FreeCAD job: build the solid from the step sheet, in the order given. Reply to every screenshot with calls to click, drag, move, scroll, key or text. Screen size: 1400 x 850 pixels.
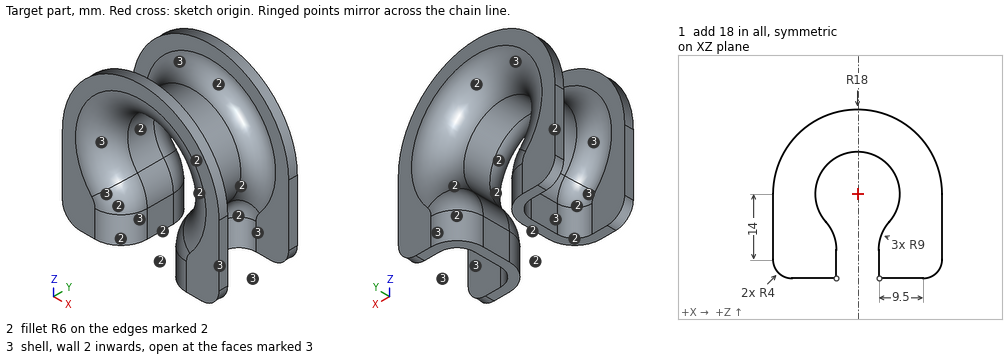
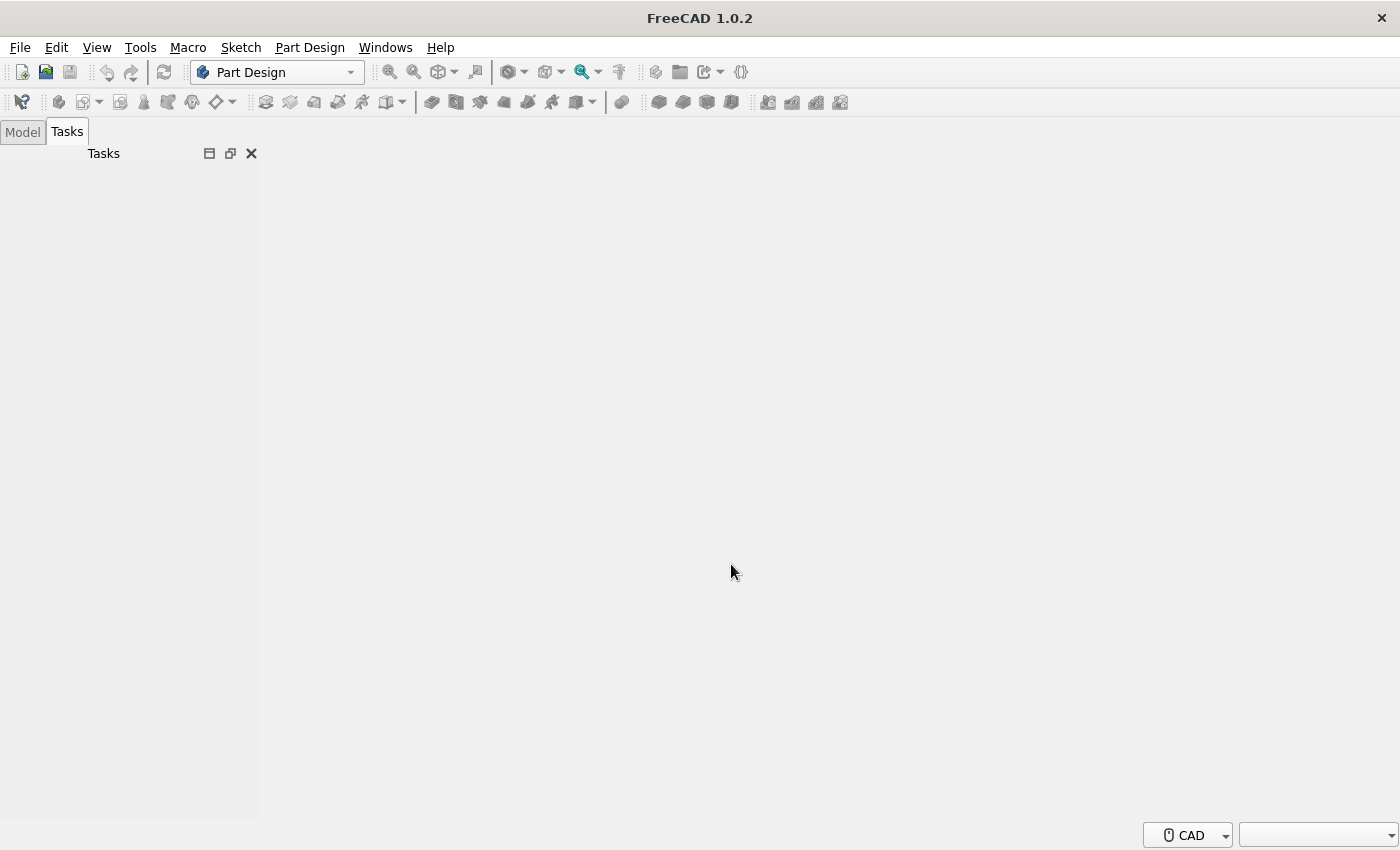
click(22, 72)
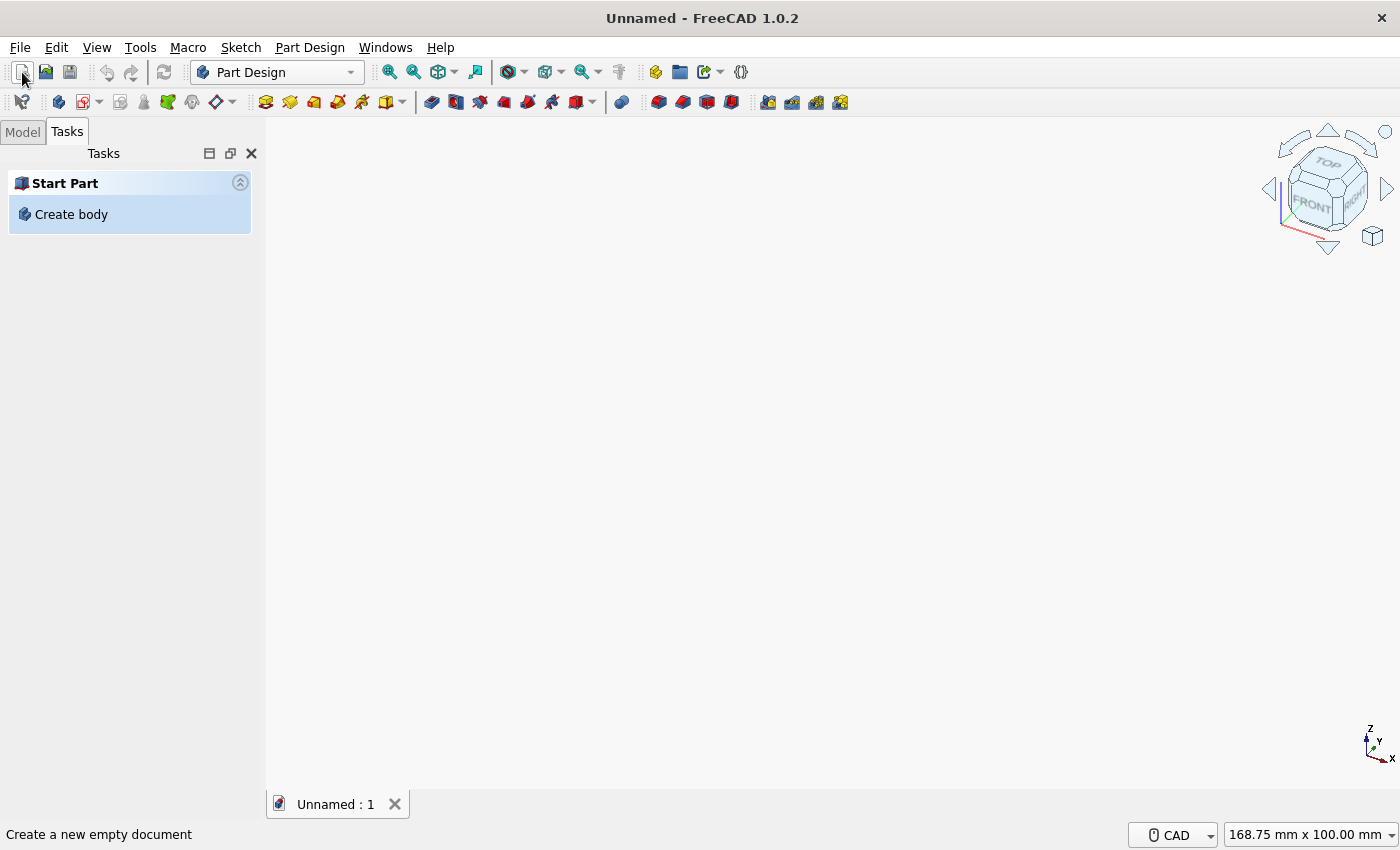
click(84, 102)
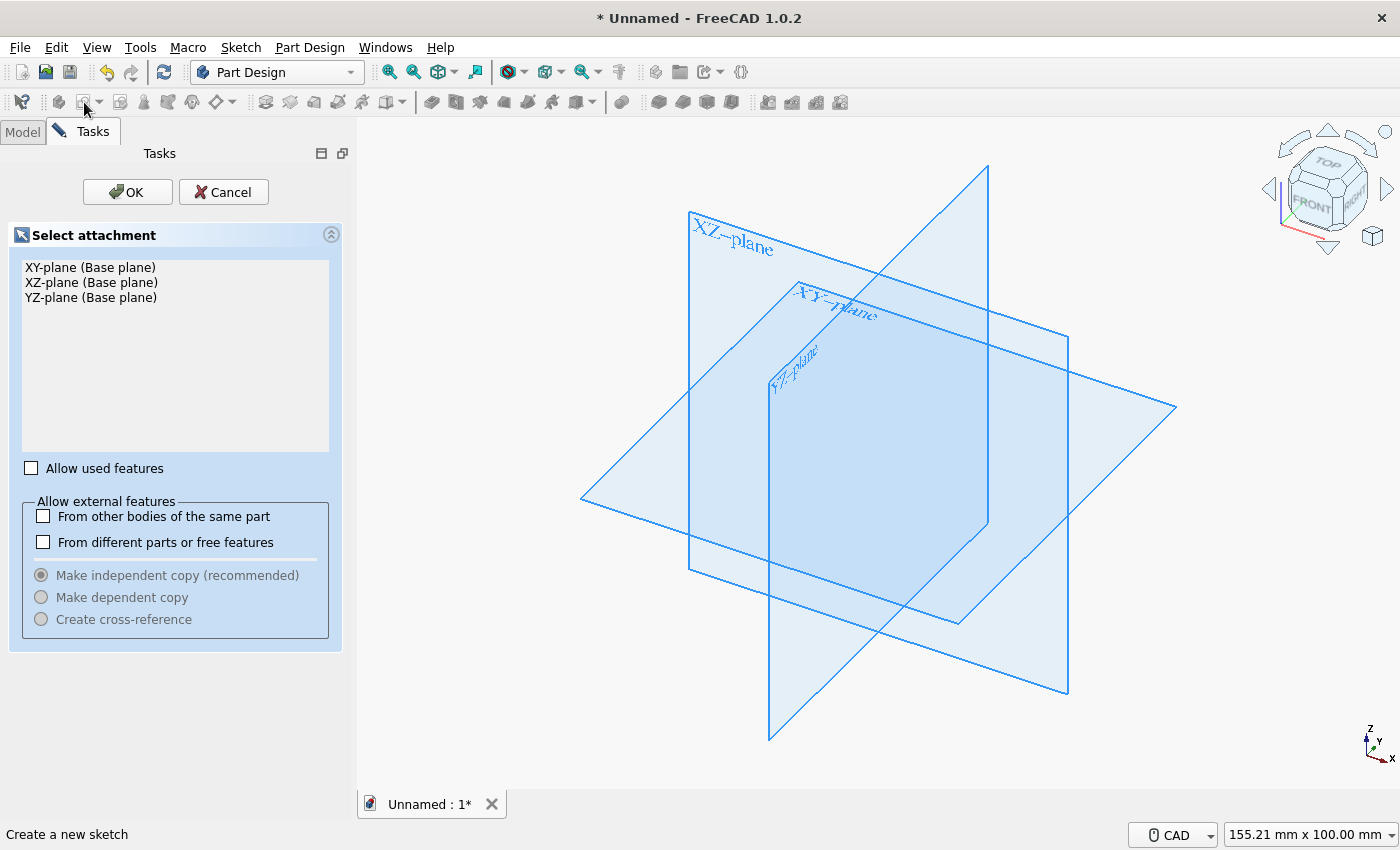
click(82, 282)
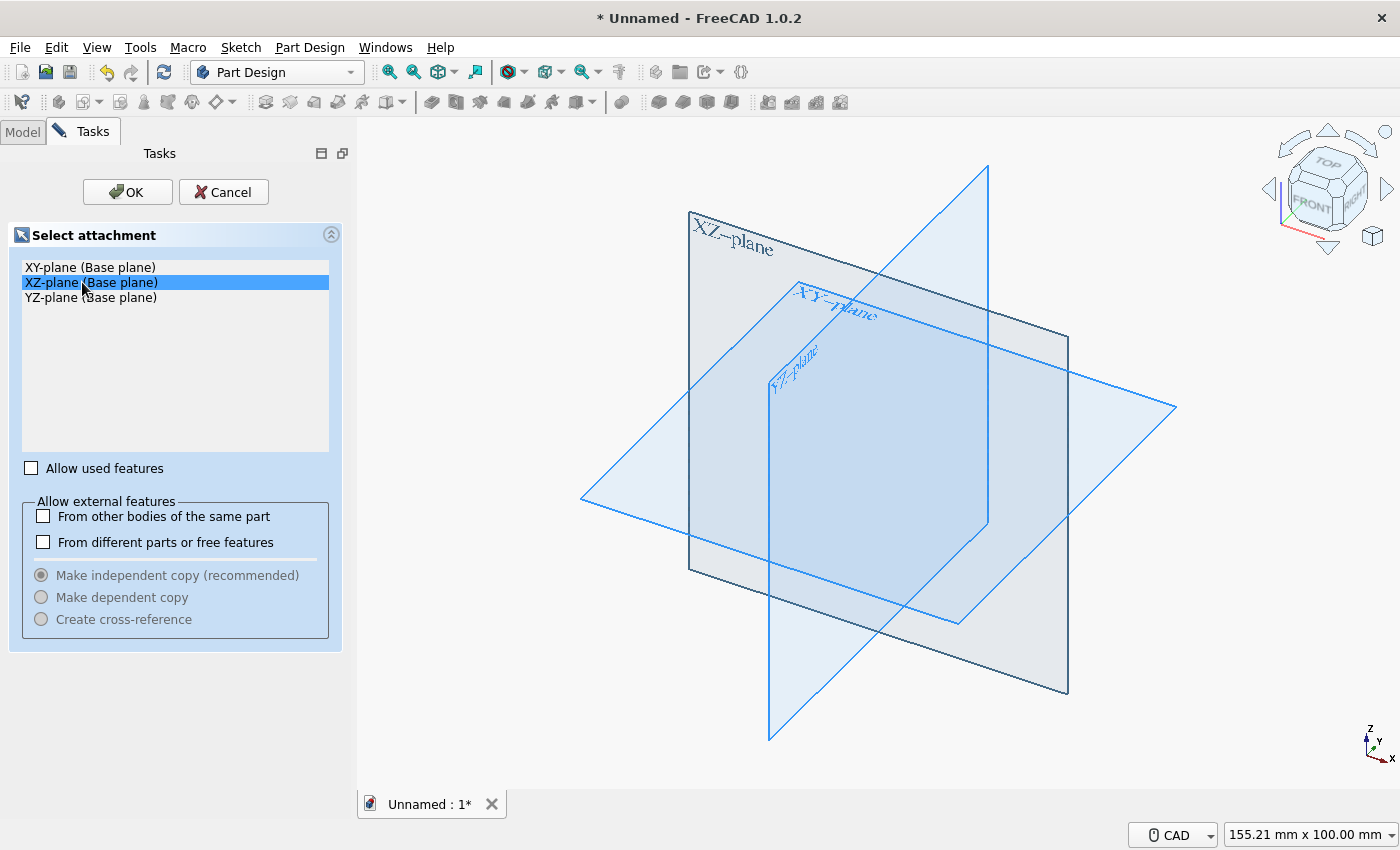
click(128, 192)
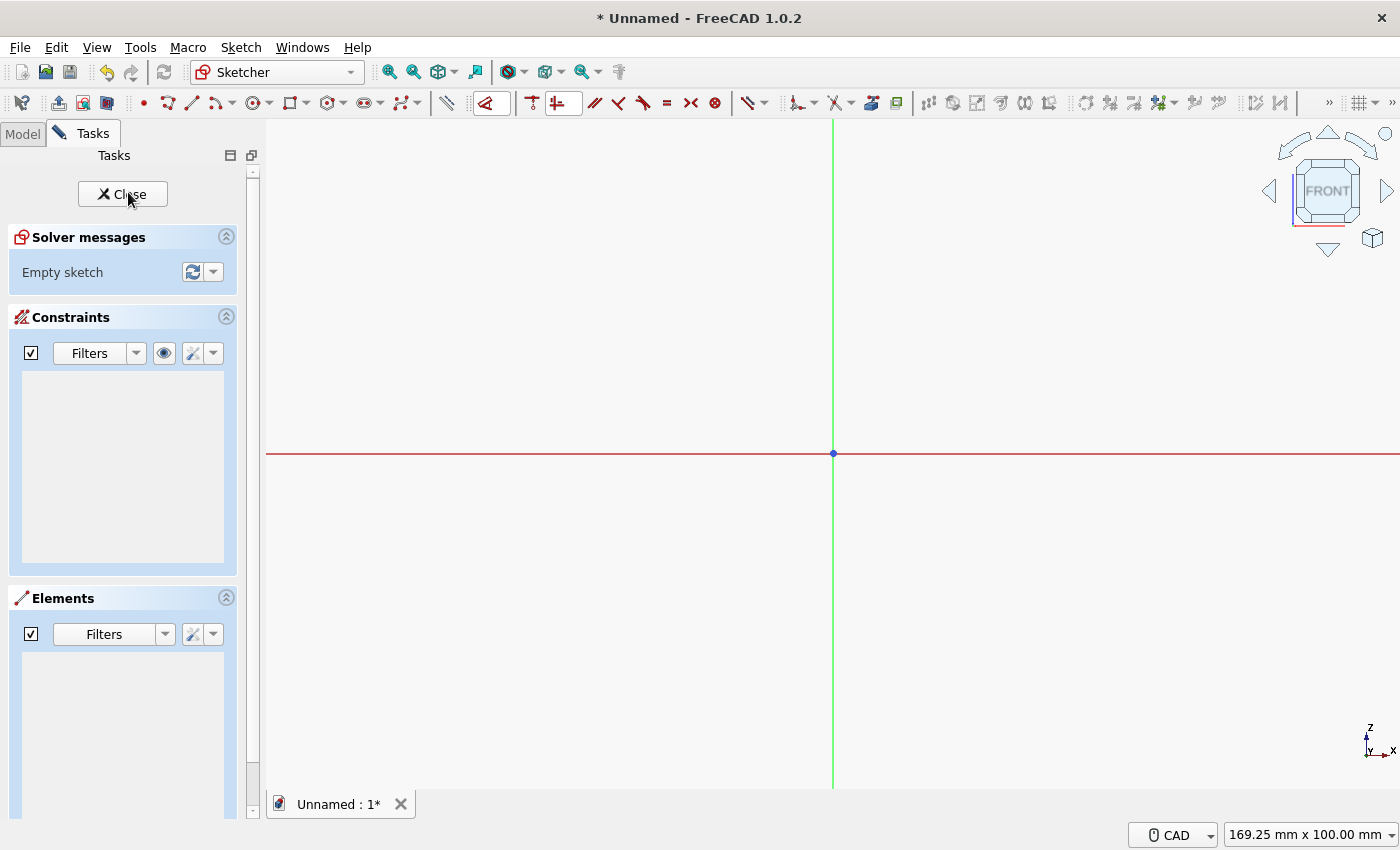
scroll(916, 454, up, 3)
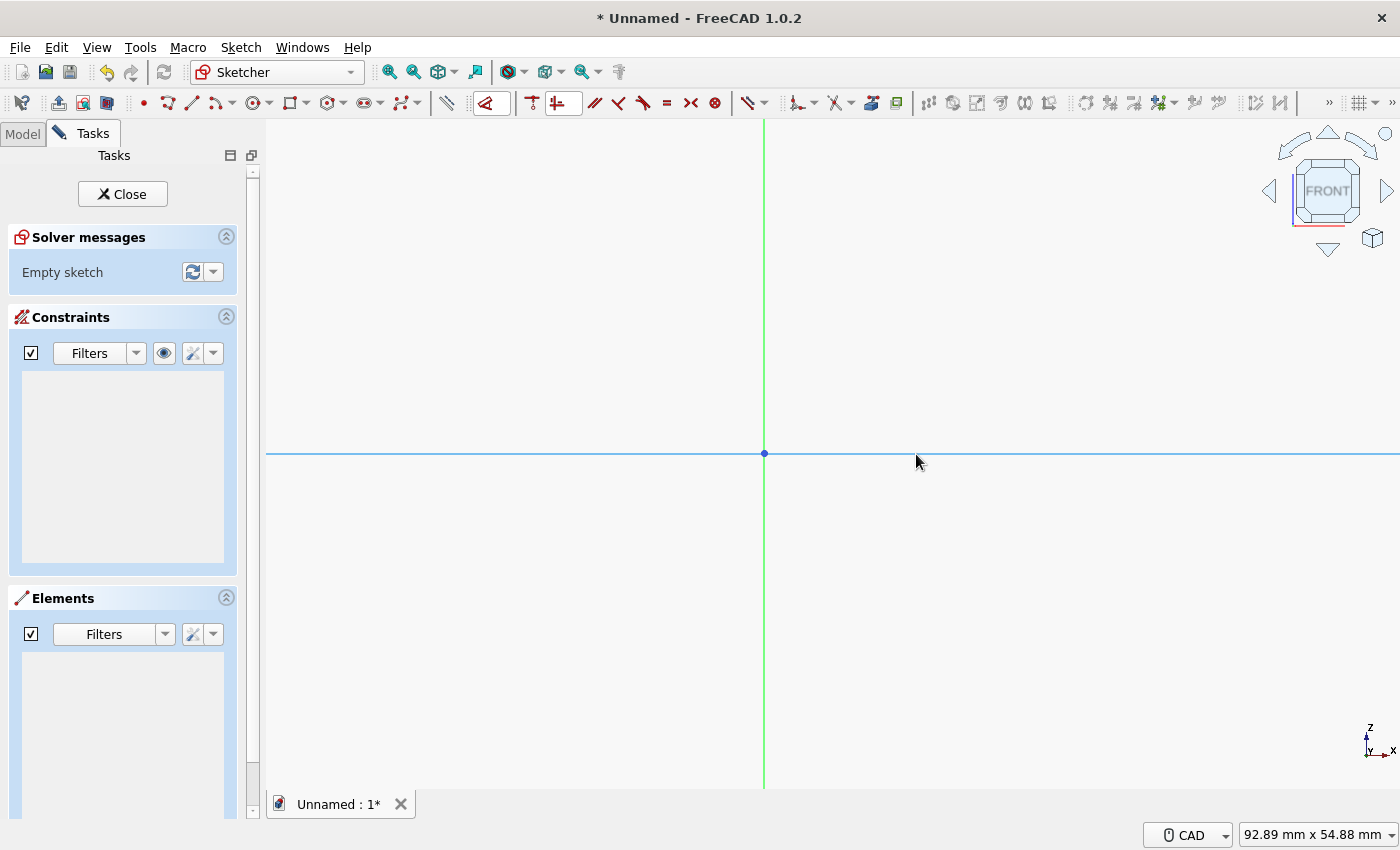
key(g)
key(l)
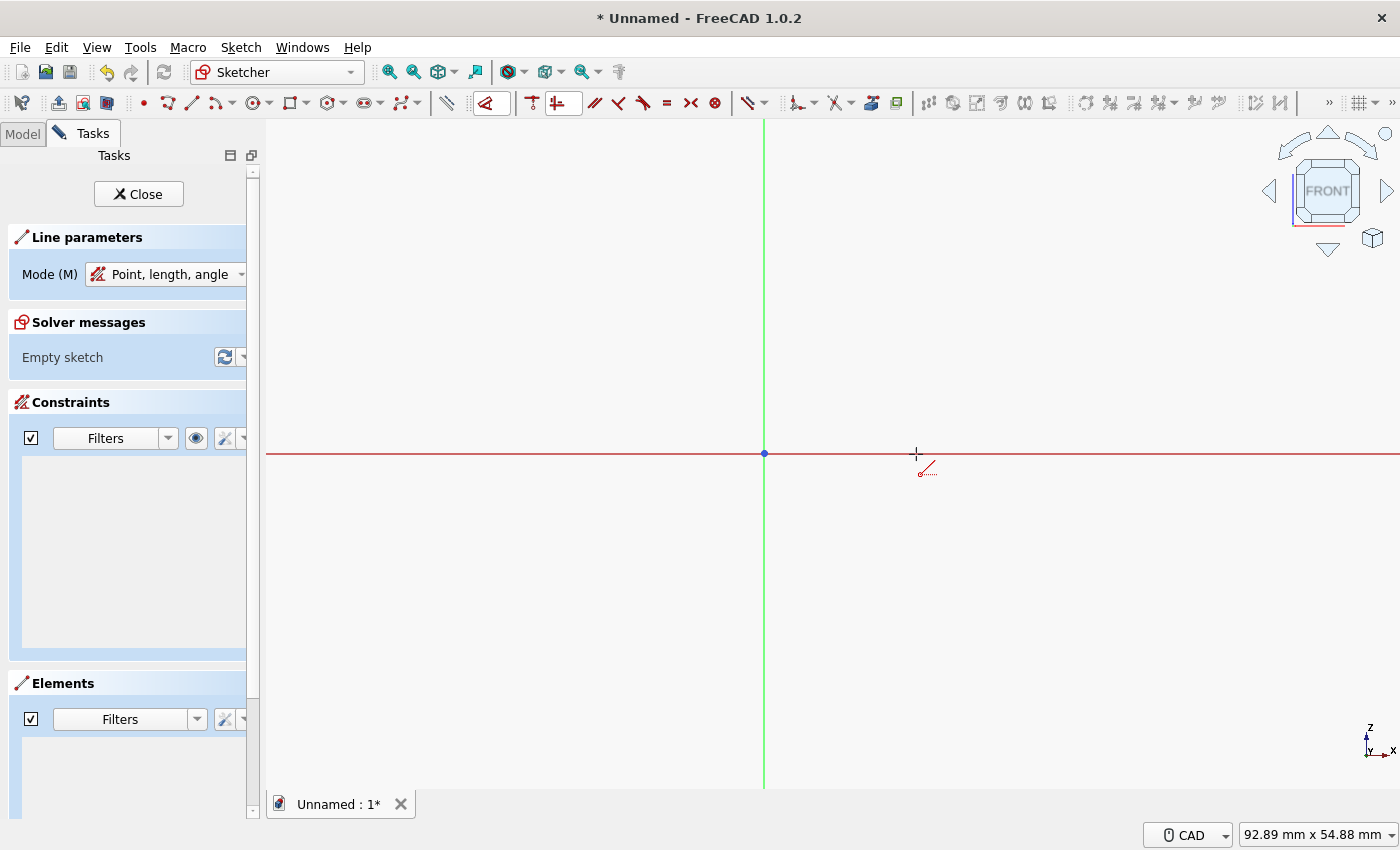
click(545, 625)
click(545, 454)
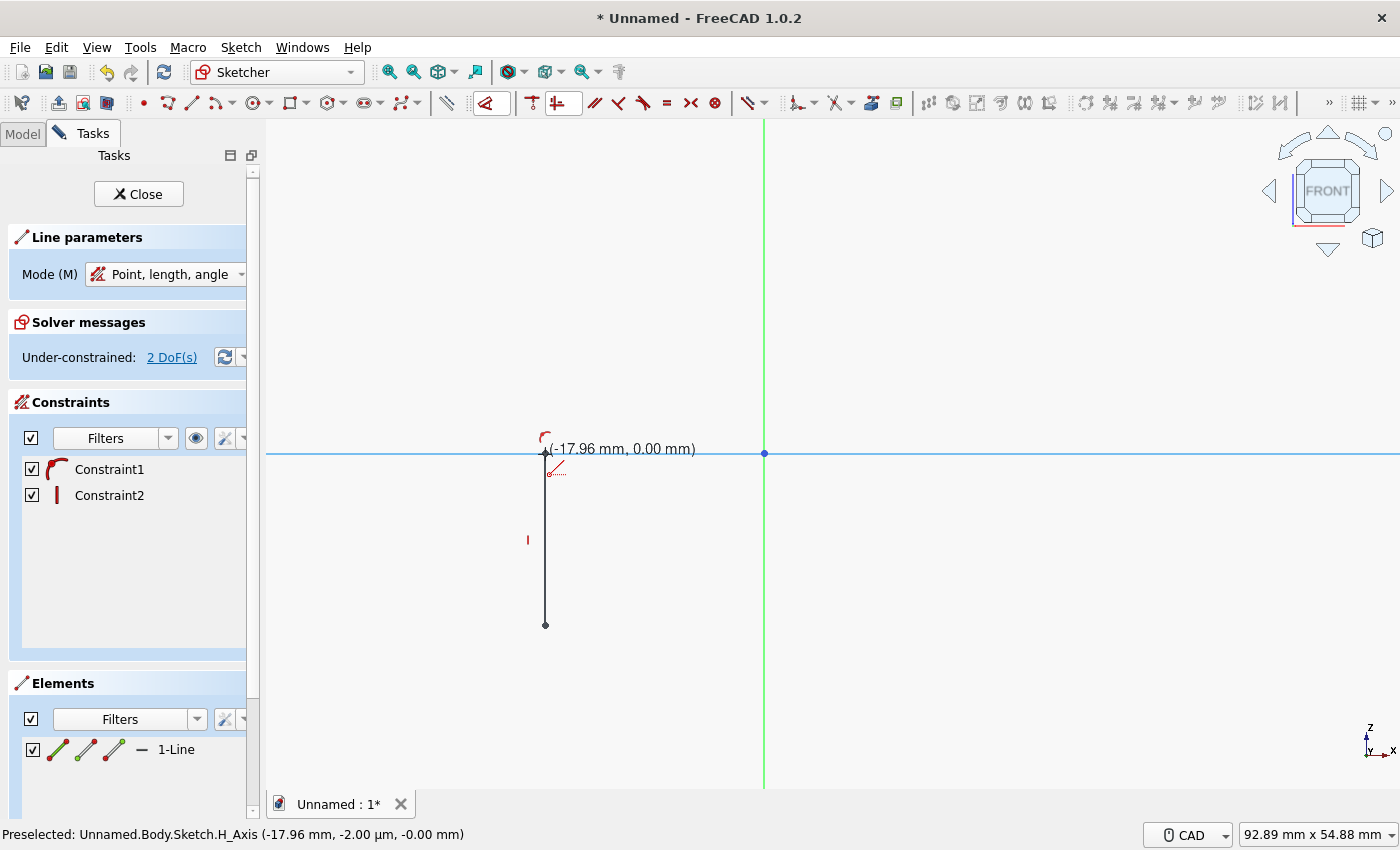
click(984, 454)
click(984, 625)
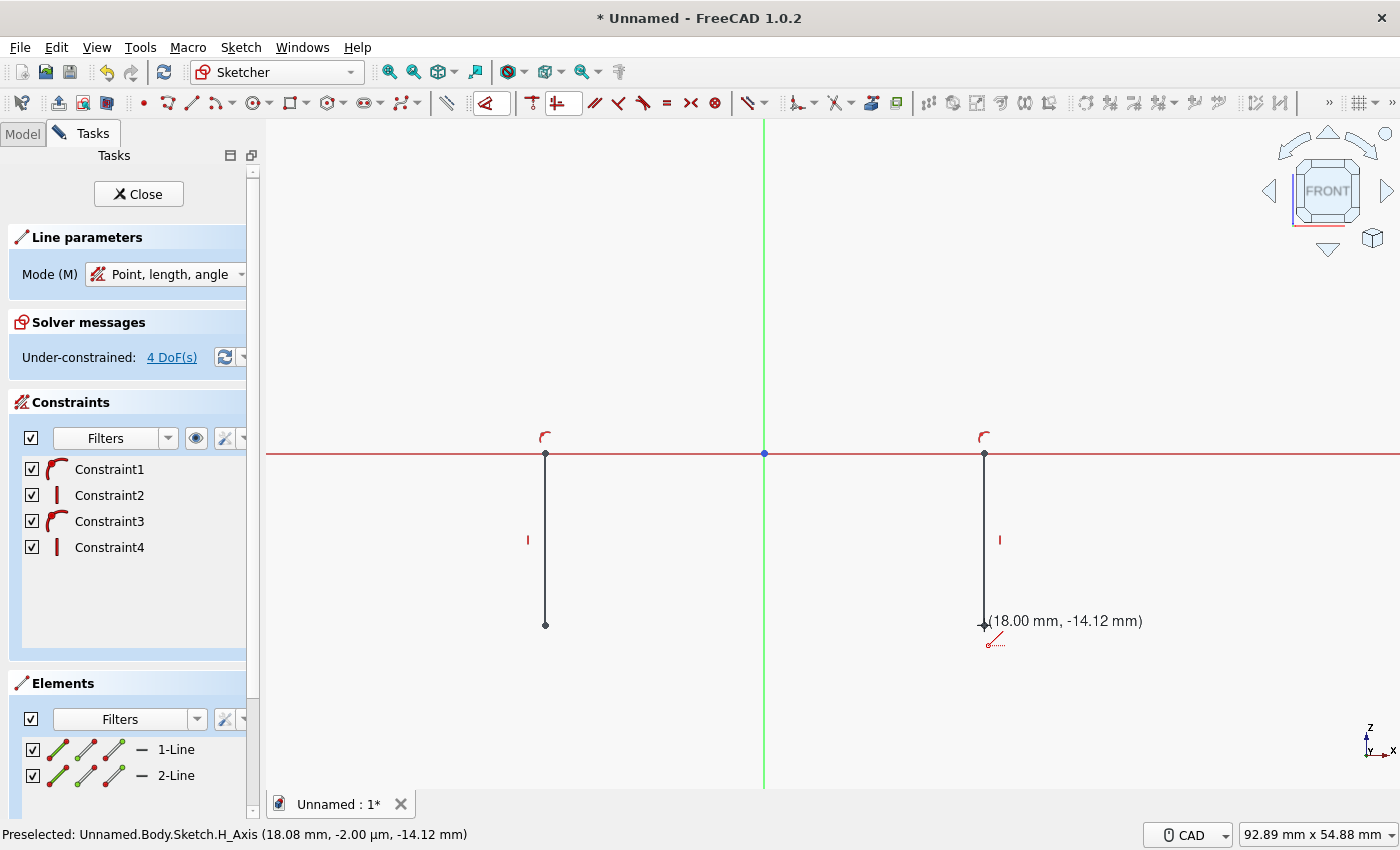
key(g)
key(m)